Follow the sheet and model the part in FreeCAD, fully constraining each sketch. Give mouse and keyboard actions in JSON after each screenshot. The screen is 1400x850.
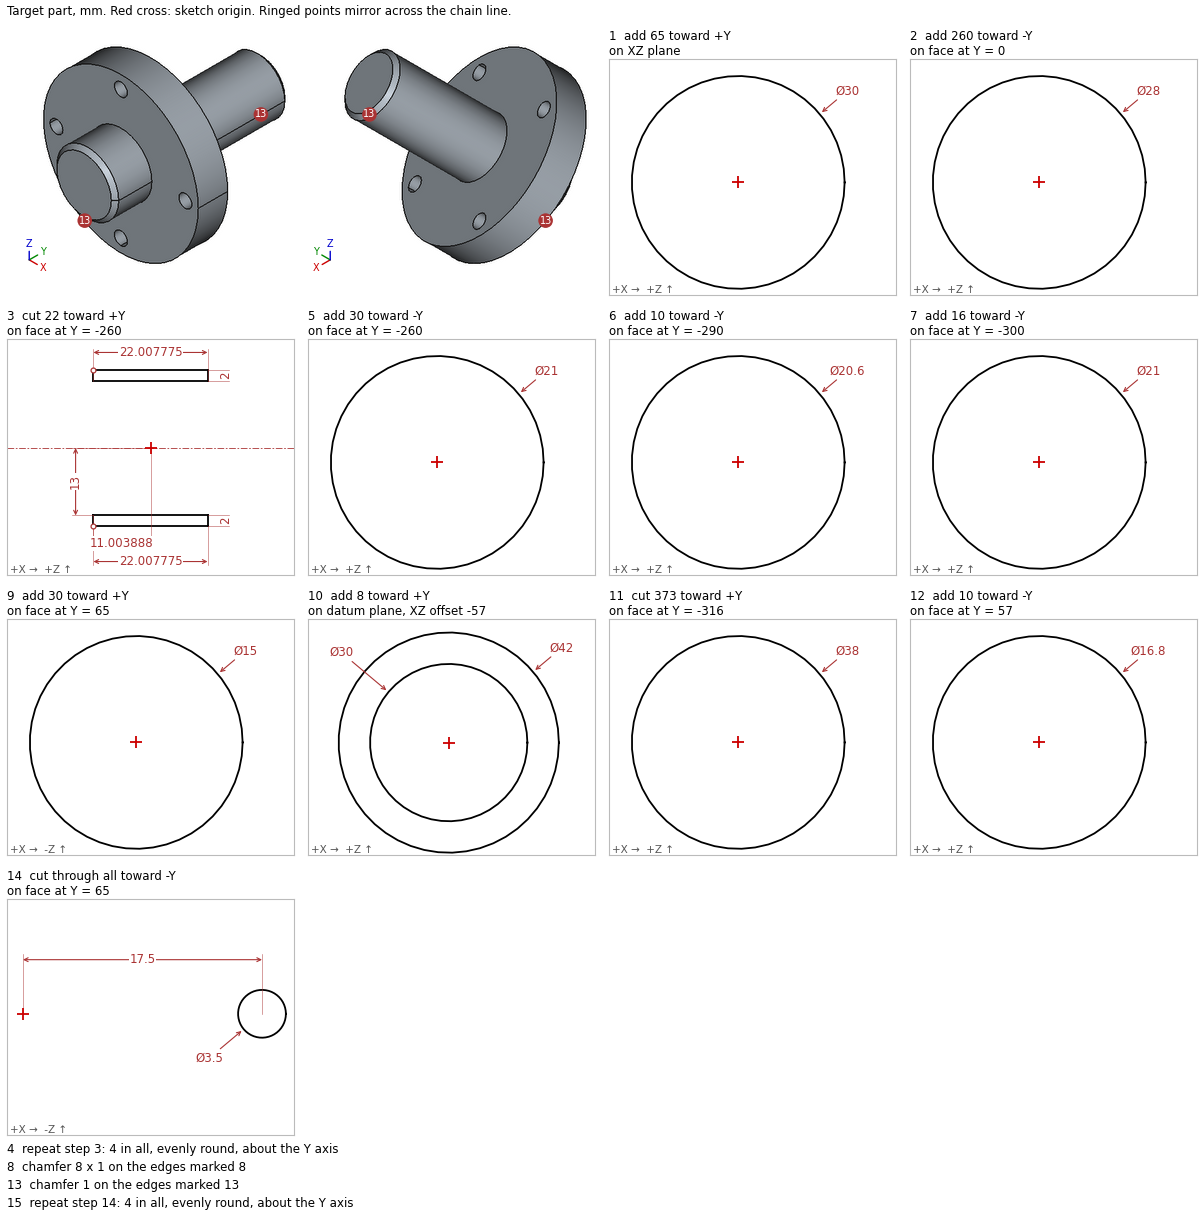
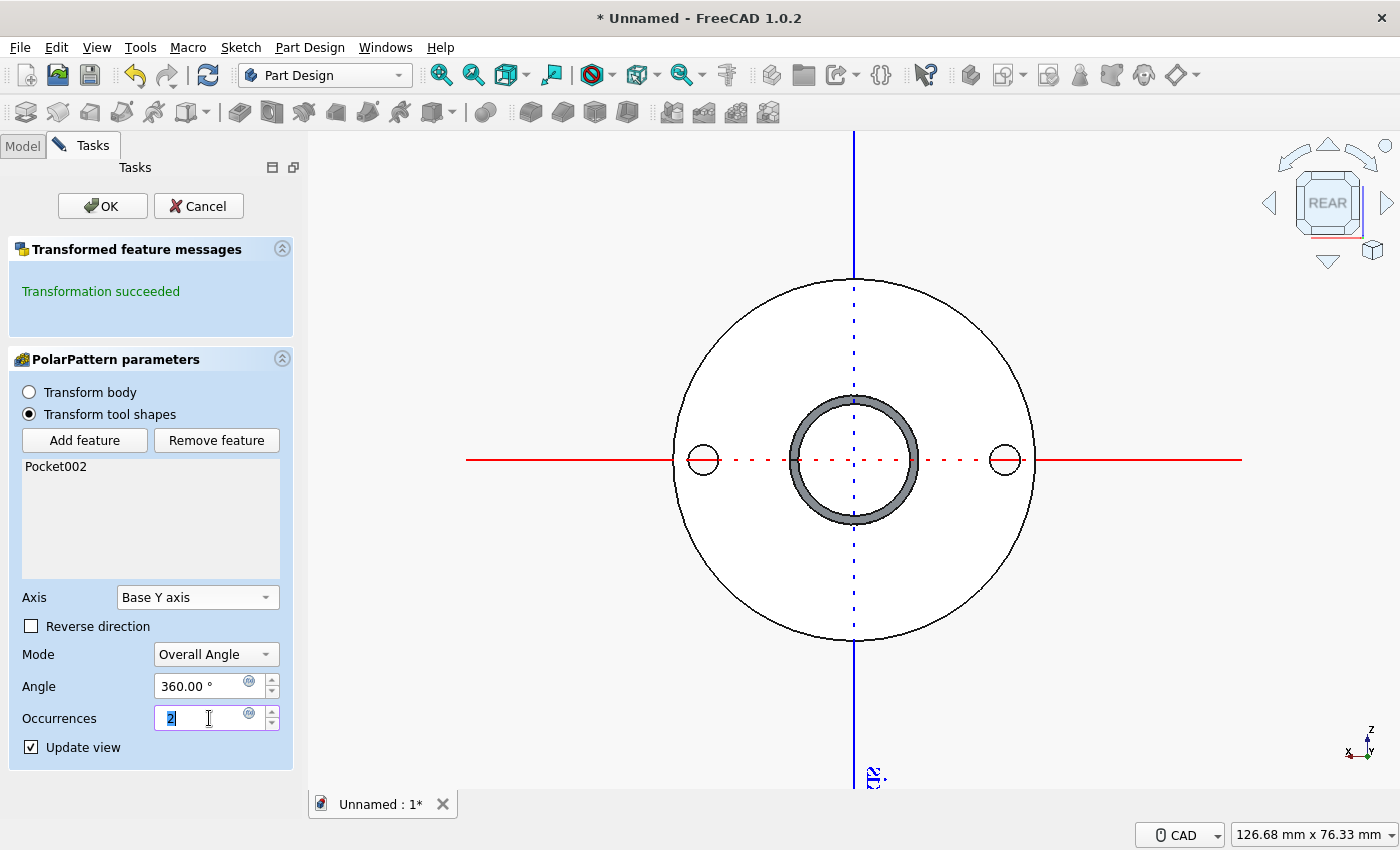
{"action": "type", "text": "4"}
{"action": "key", "text": "Tab"}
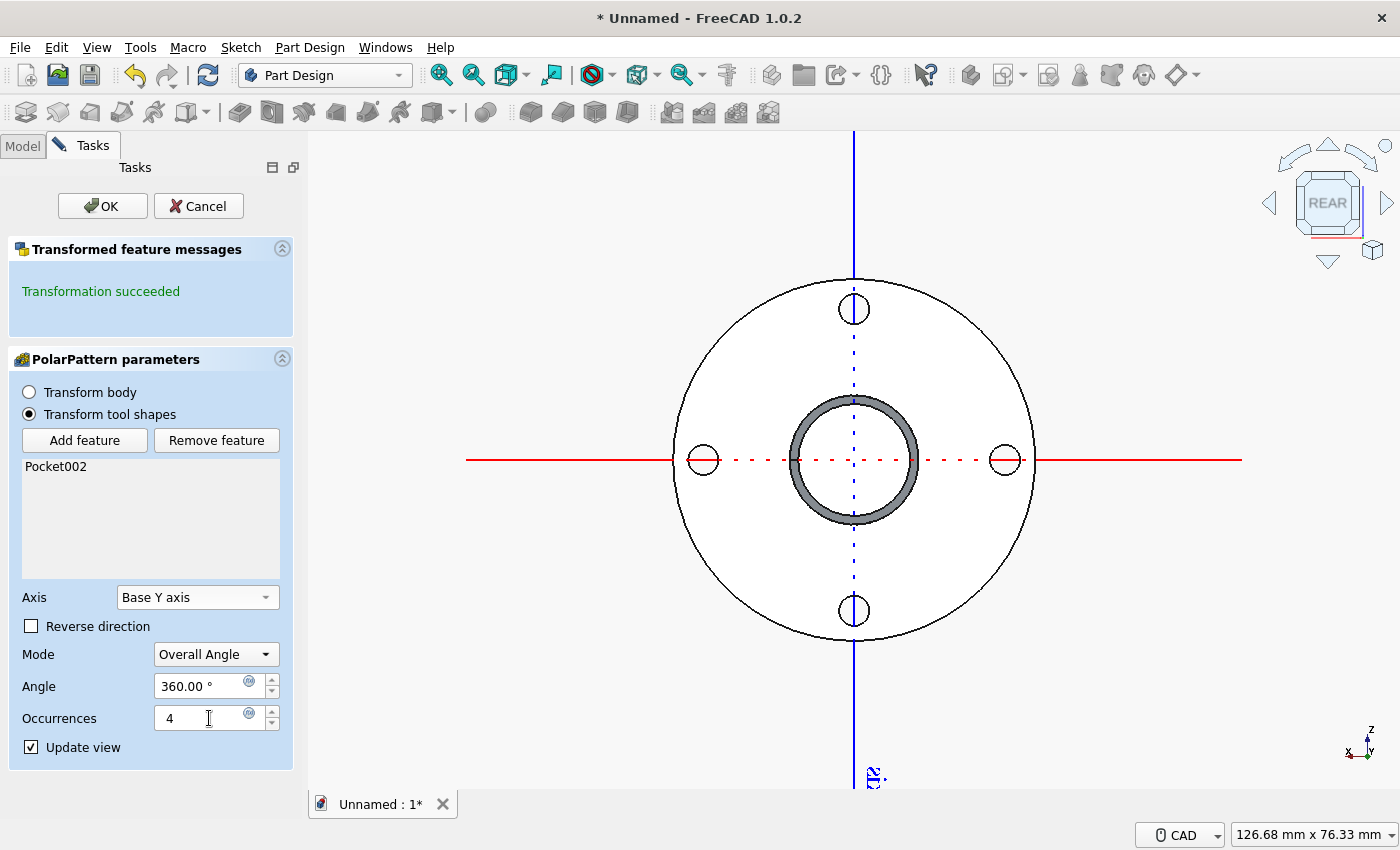
{"action": "left_click", "coordinate": [103, 206]}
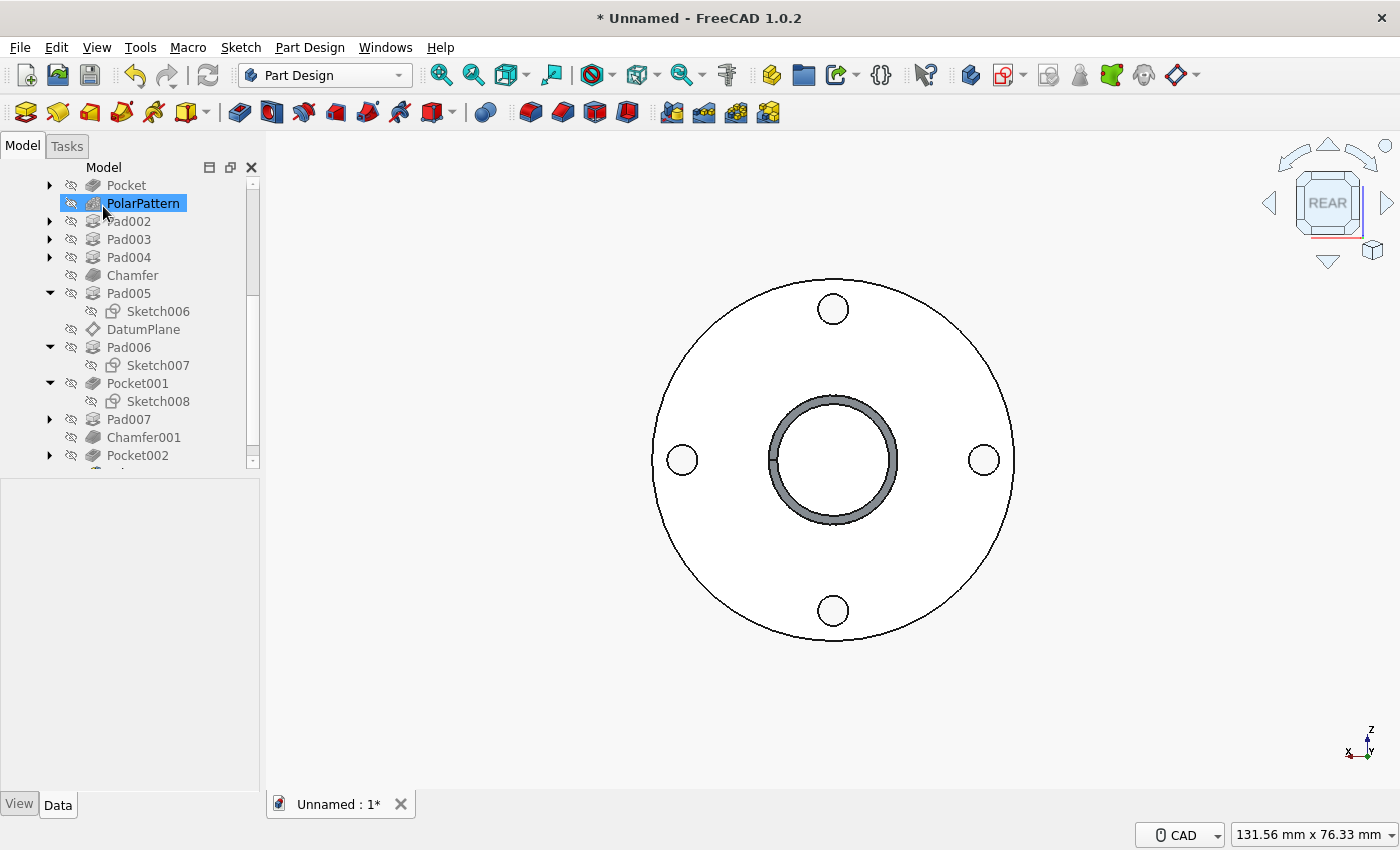
{"action": "key", "text": "0"}